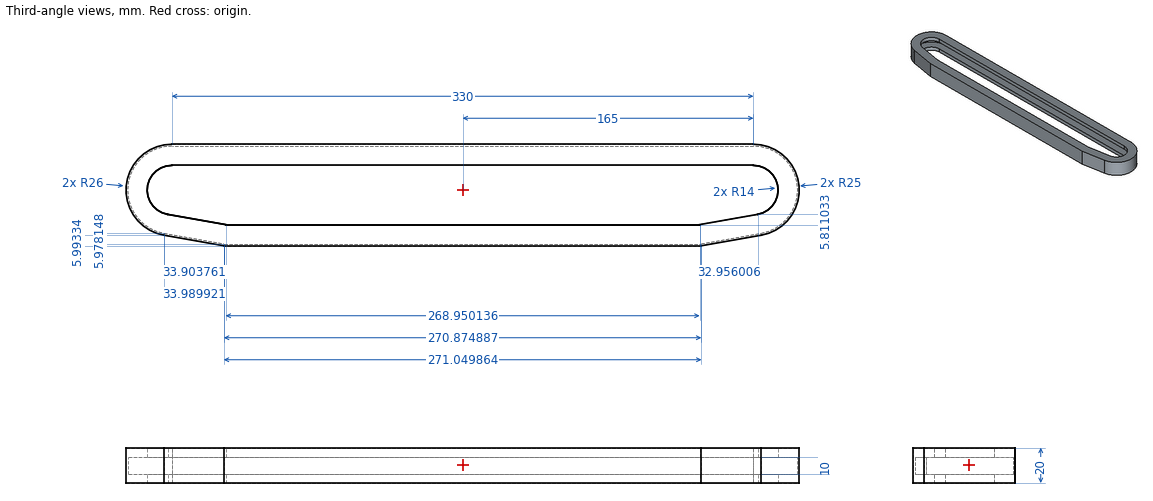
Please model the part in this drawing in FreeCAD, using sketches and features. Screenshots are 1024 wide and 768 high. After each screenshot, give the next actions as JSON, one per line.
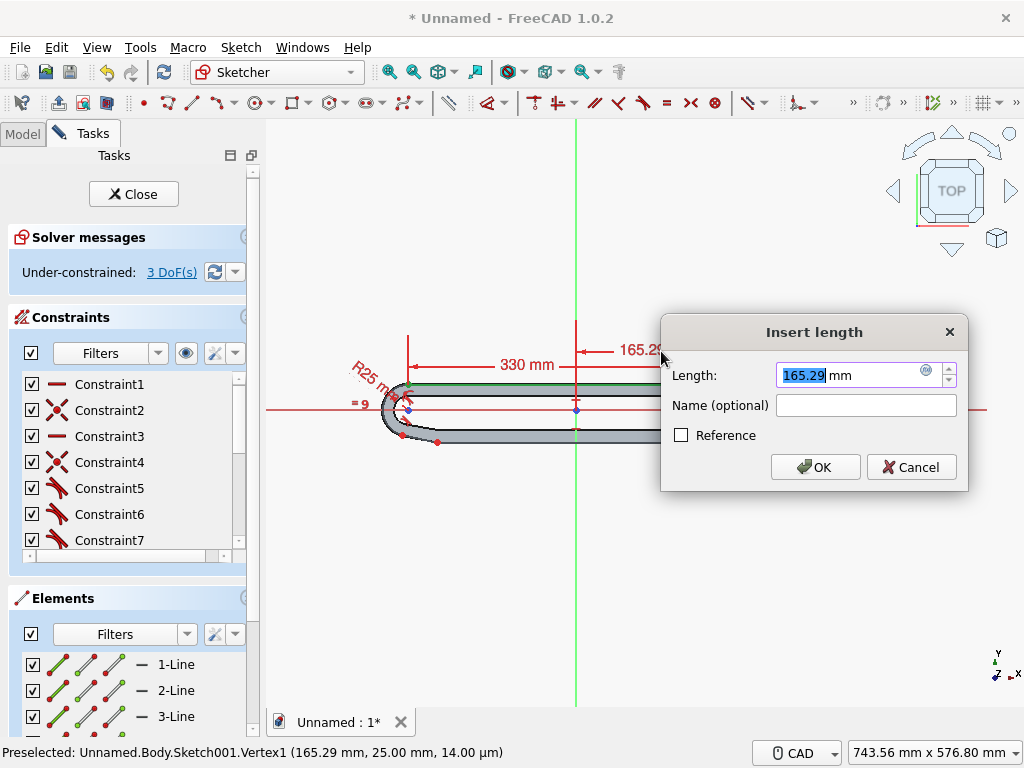
{"action": "type", "text": "165"}
{"action": "key", "text": "Return"}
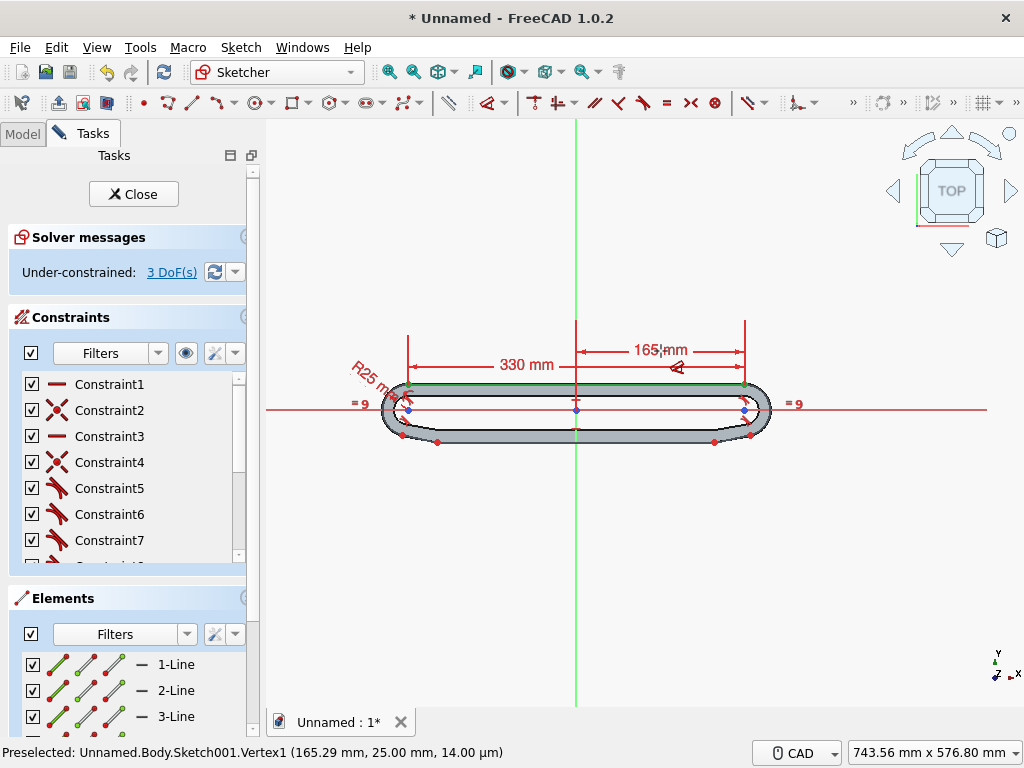
{"action": "scroll", "coordinate": [413, 438], "scroll_direction": "up", "scroll_amount": 10}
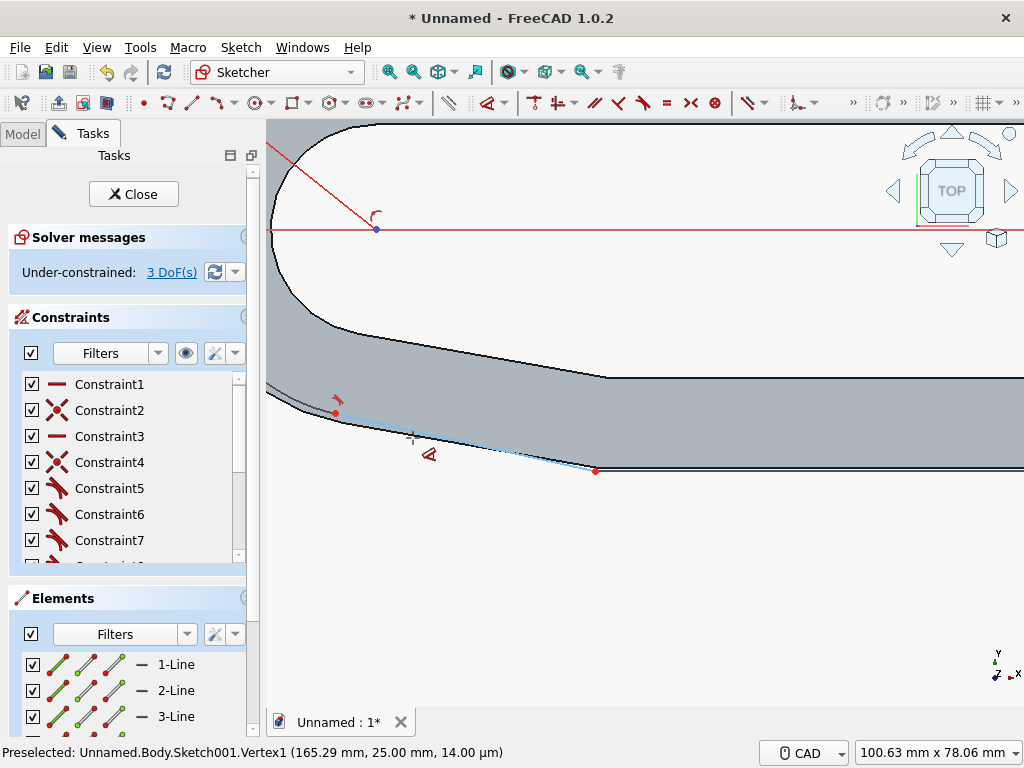
{"action": "left_click", "coordinate": [413, 431]}
{"action": "left_click", "coordinate": [301, 443]}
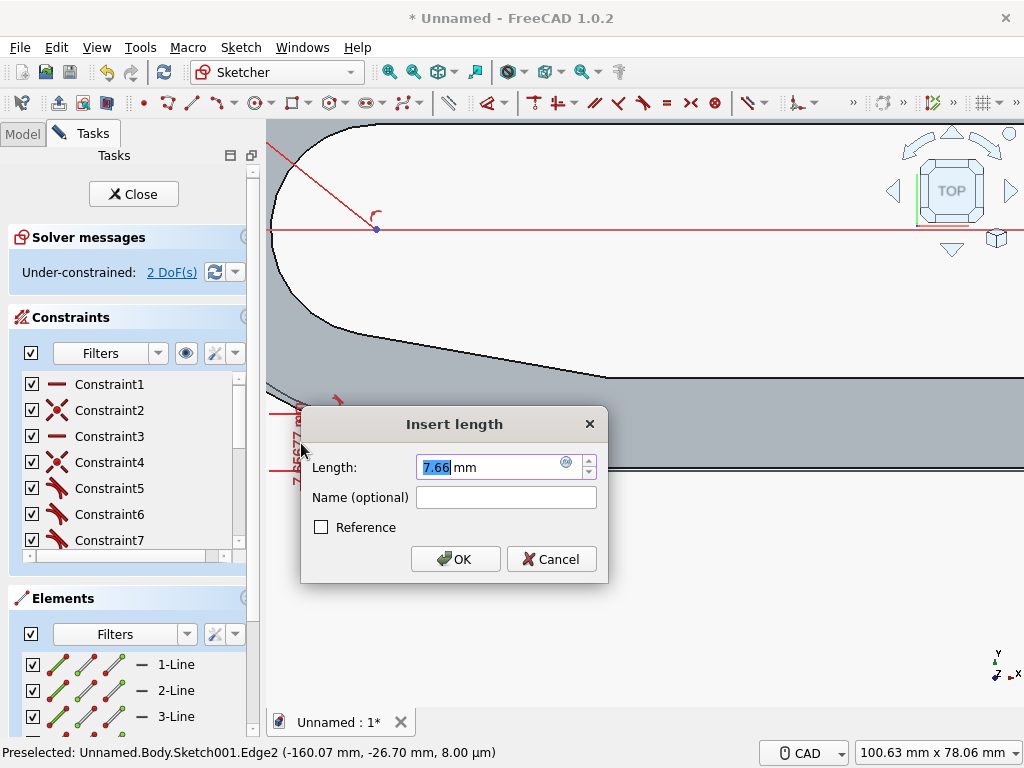
{"action": "type", "text": "5.978148"}
{"action": "key", "text": "Return"}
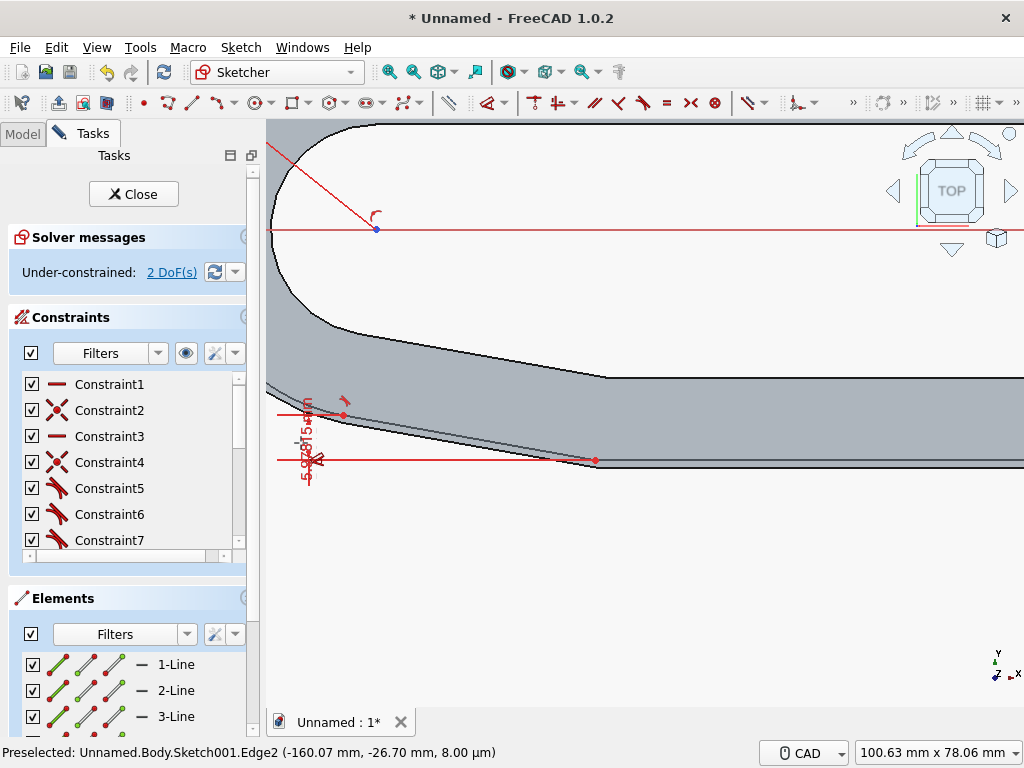
{"action": "scroll", "coordinate": [413, 438], "scroll_direction": "down", "scroll_amount": 10}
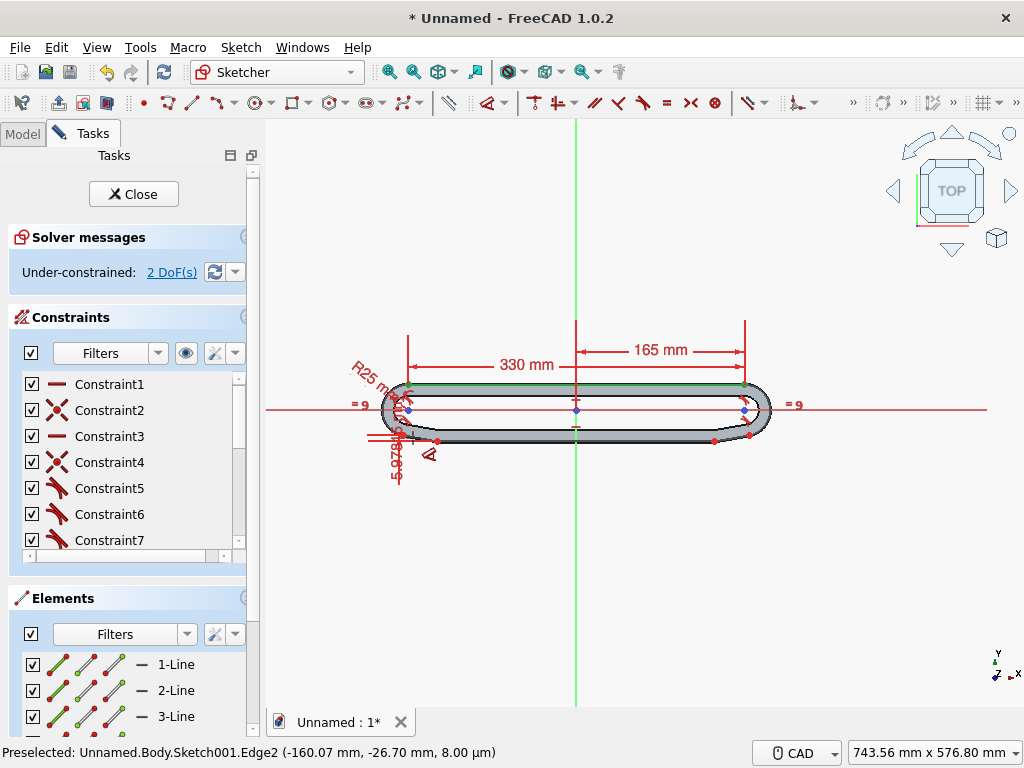
{"action": "left_click", "coordinate": [521, 441]}
{"action": "left_click", "coordinate": [513, 475]}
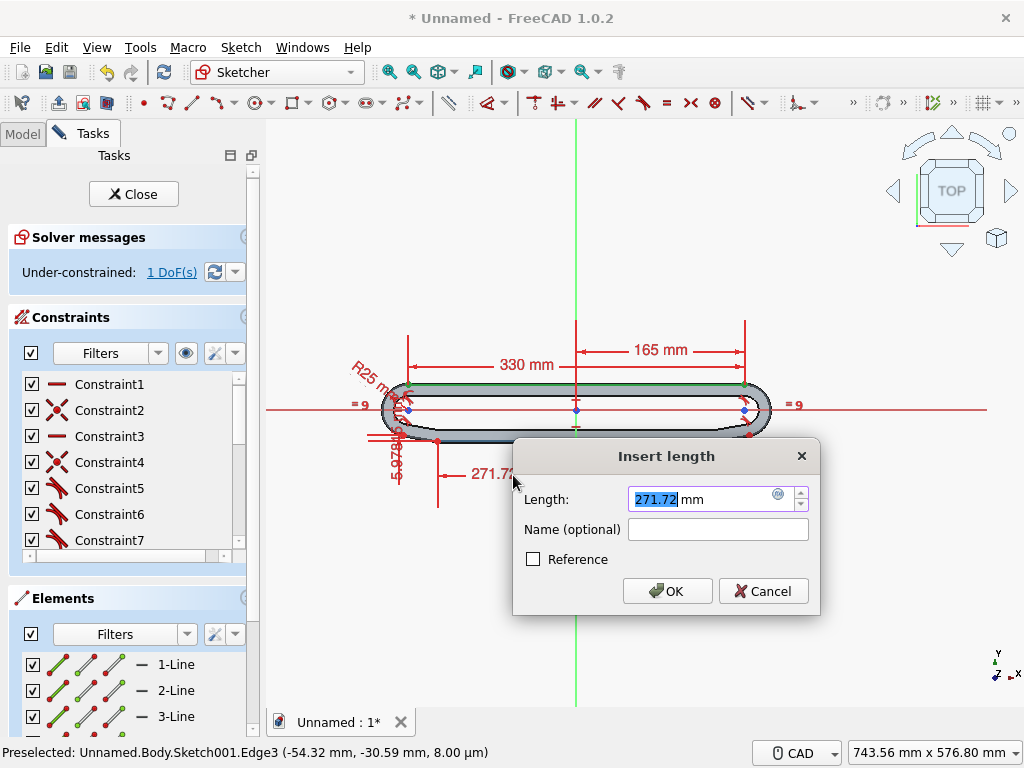
{"action": "type", "text": "270.874887"}
{"action": "key", "text": "Return"}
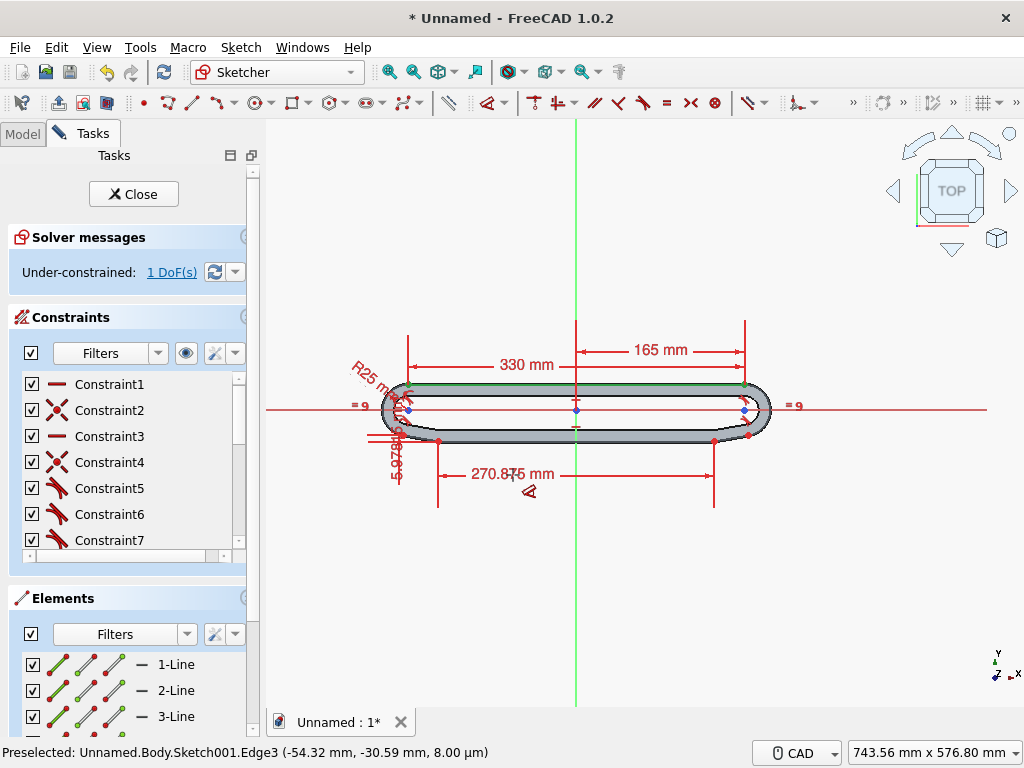
{"action": "scroll", "coordinate": [414, 437], "scroll_direction": "up", "scroll_amount": 2}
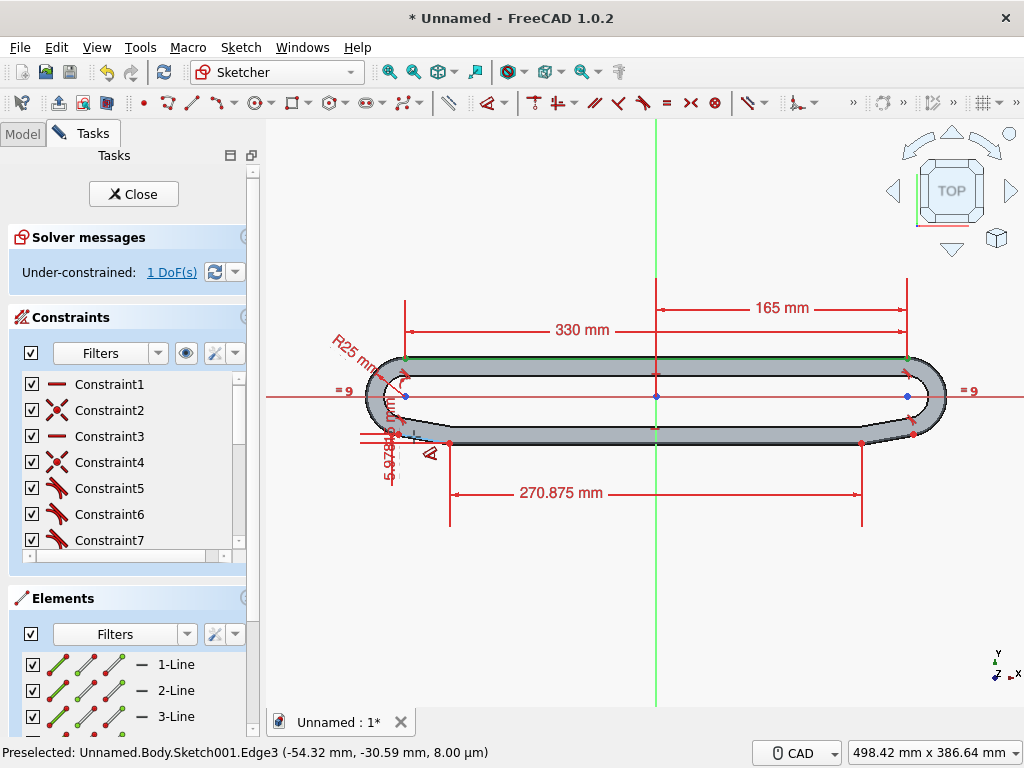
{"action": "left_click", "coordinate": [414, 437]}
{"action": "left_click", "coordinate": [424, 477]}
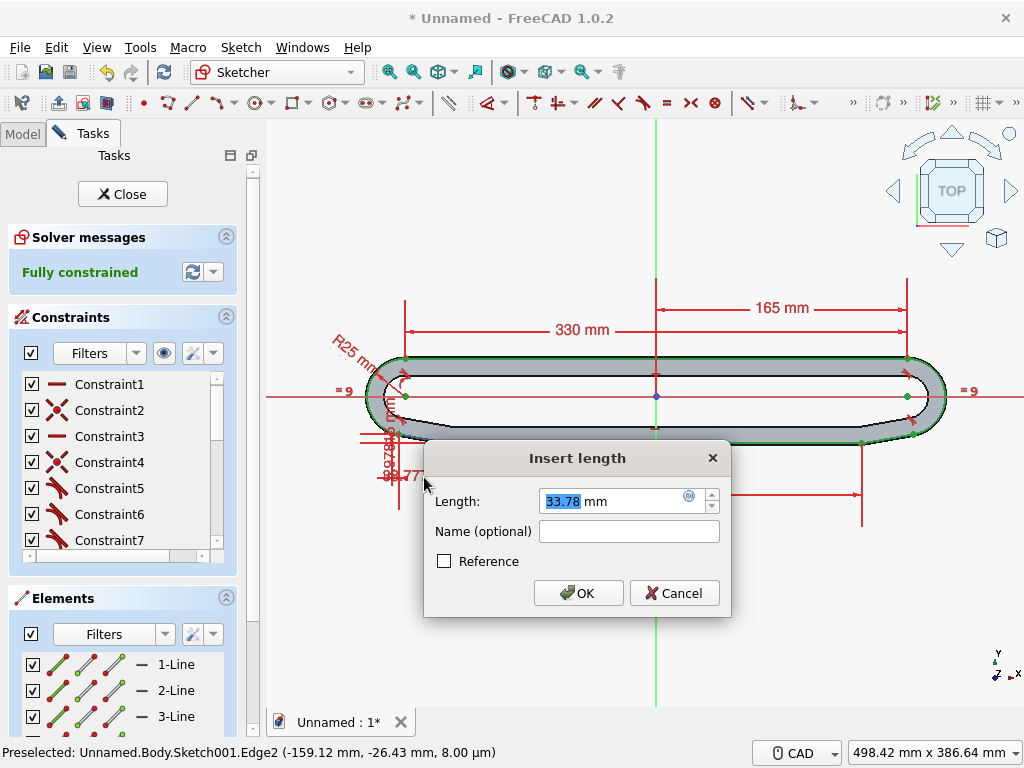
{"action": "type", "text": "33.903761"}
{"action": "key", "text": "Return"}
{"action": "key", "text": "Escape"}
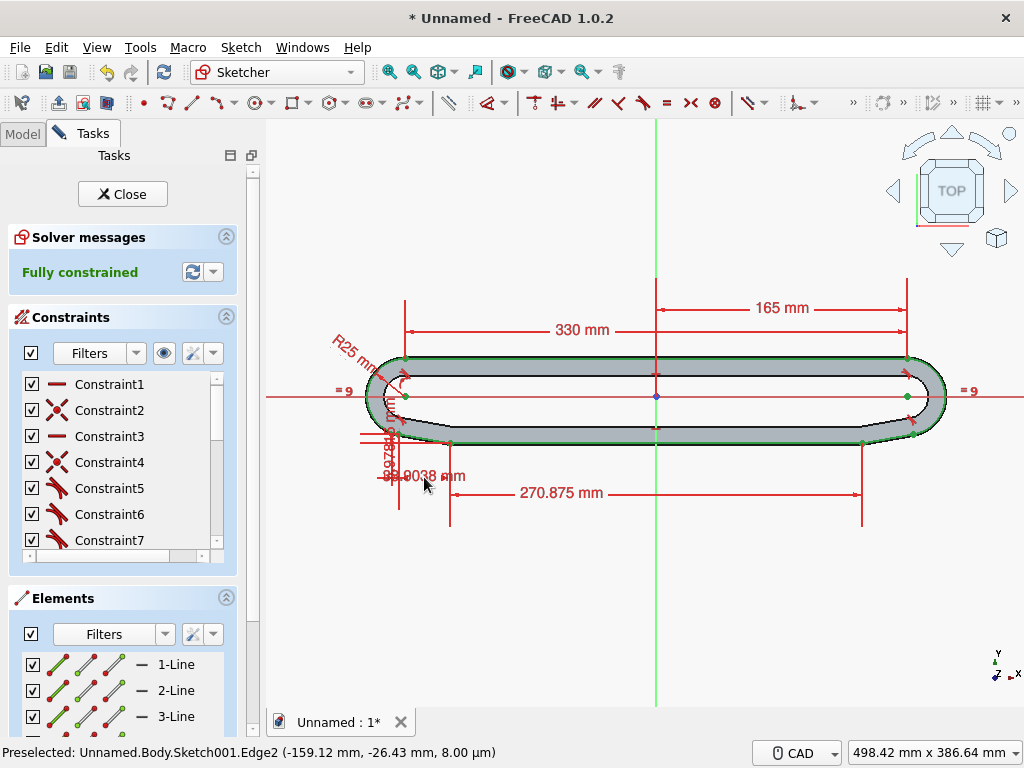
{"action": "left_click", "coordinate": [123, 194]}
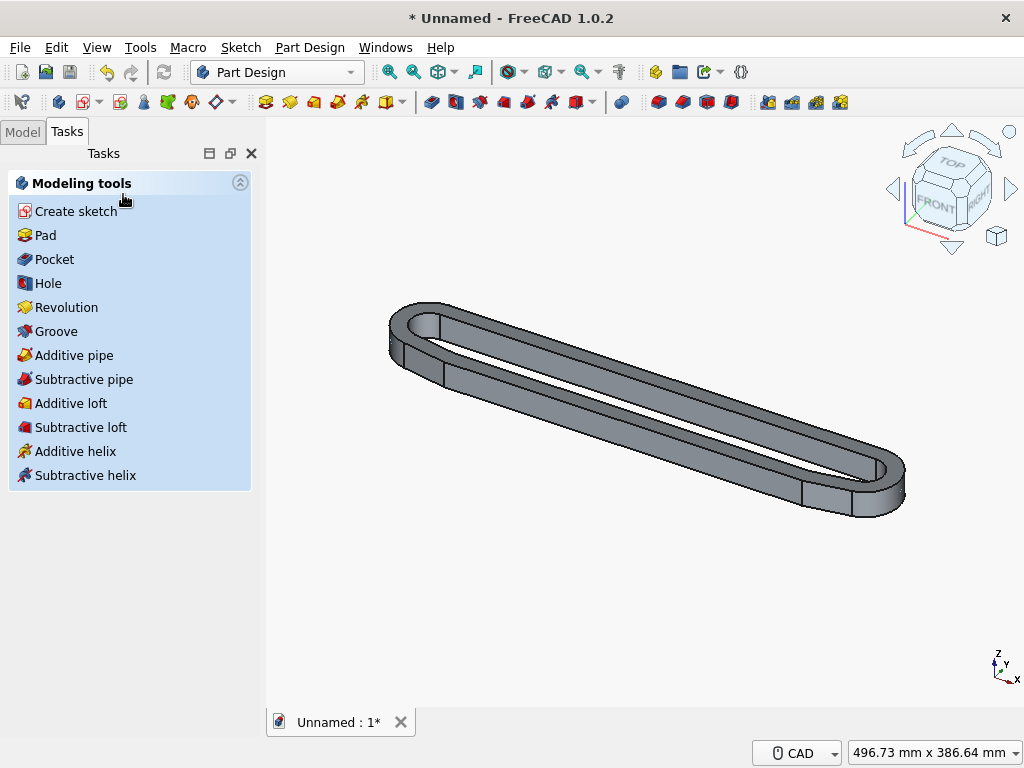
{"action": "left_click", "coordinate": [432, 102]}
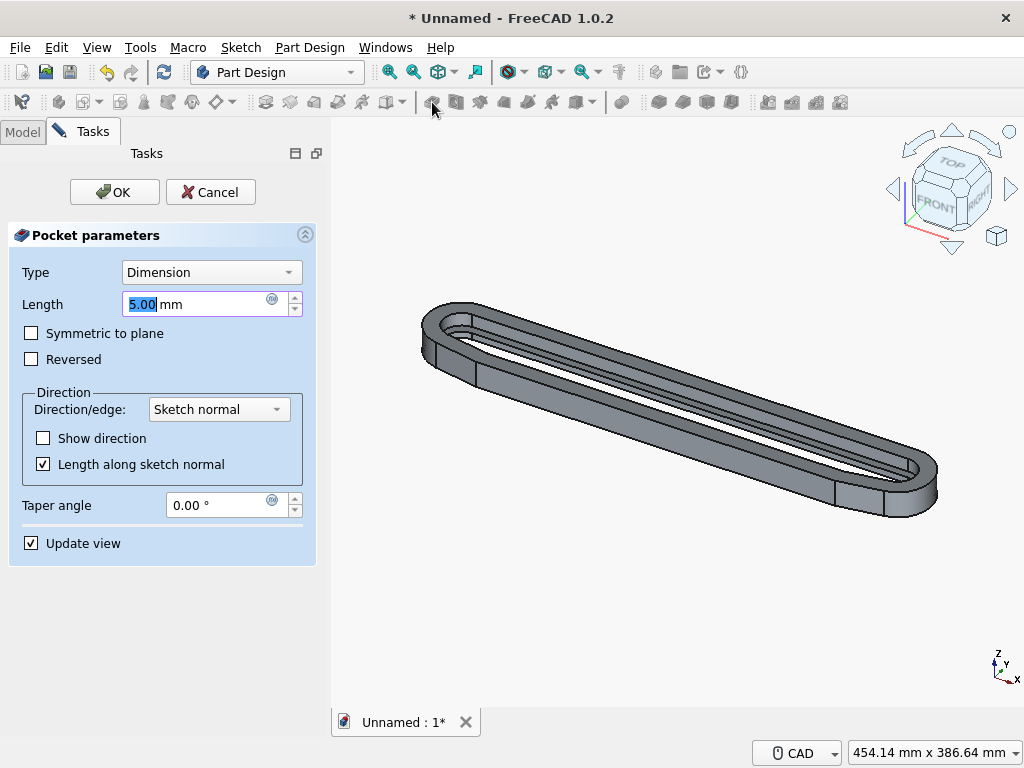
{"action": "type", "text": "10"}
{"action": "key", "text": "Tab"}